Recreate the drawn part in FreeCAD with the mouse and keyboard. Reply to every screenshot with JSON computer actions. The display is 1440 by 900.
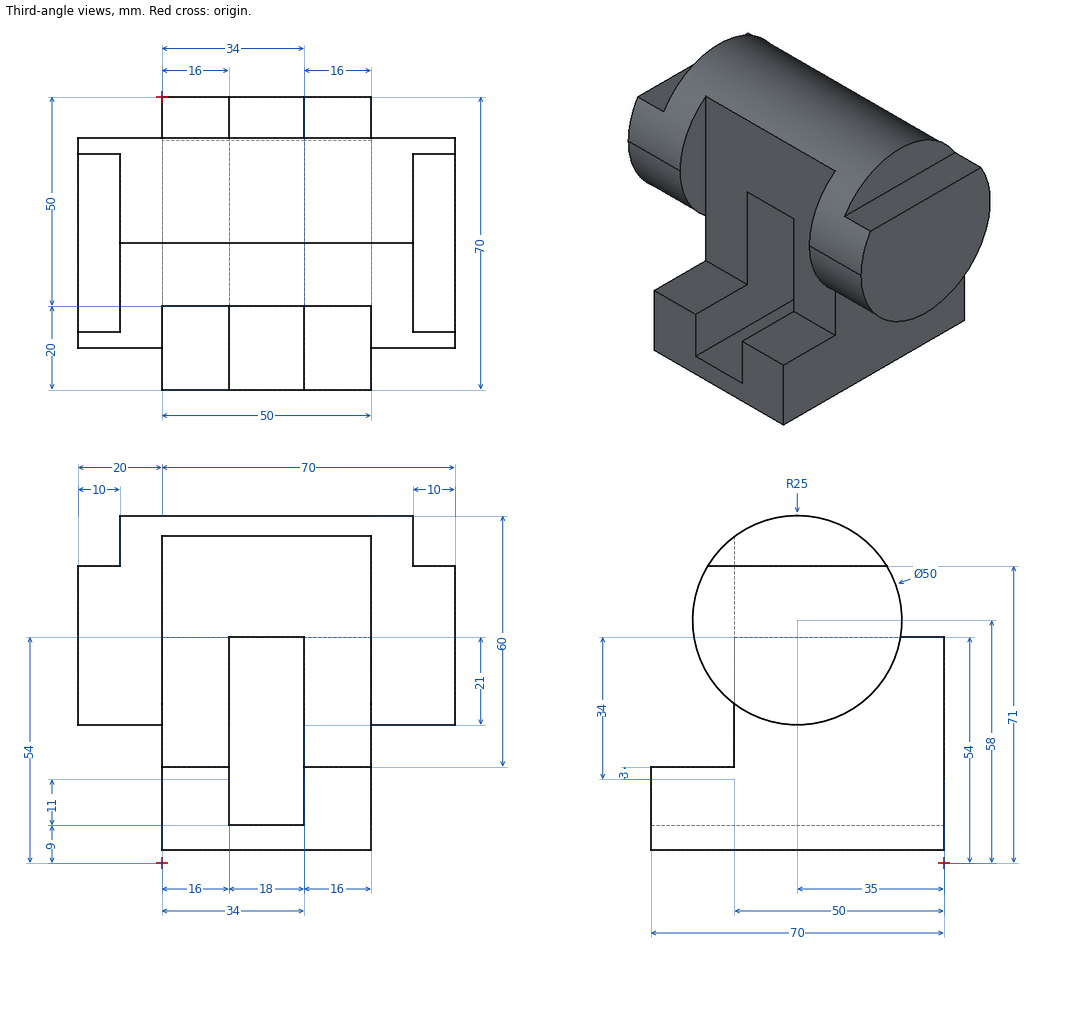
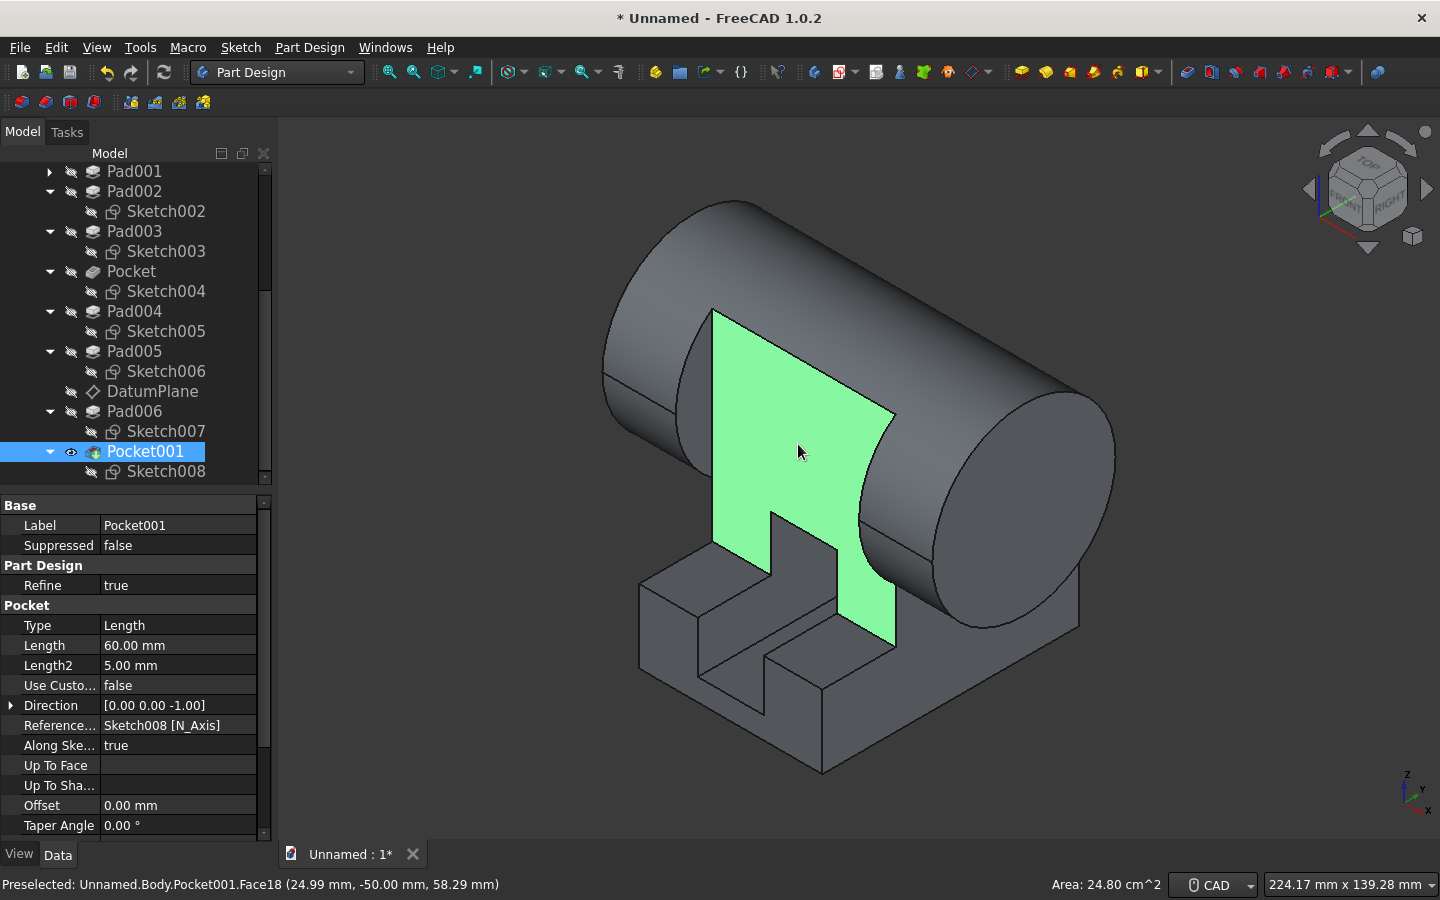
{"action": "left_click", "coordinate": [840, 72]}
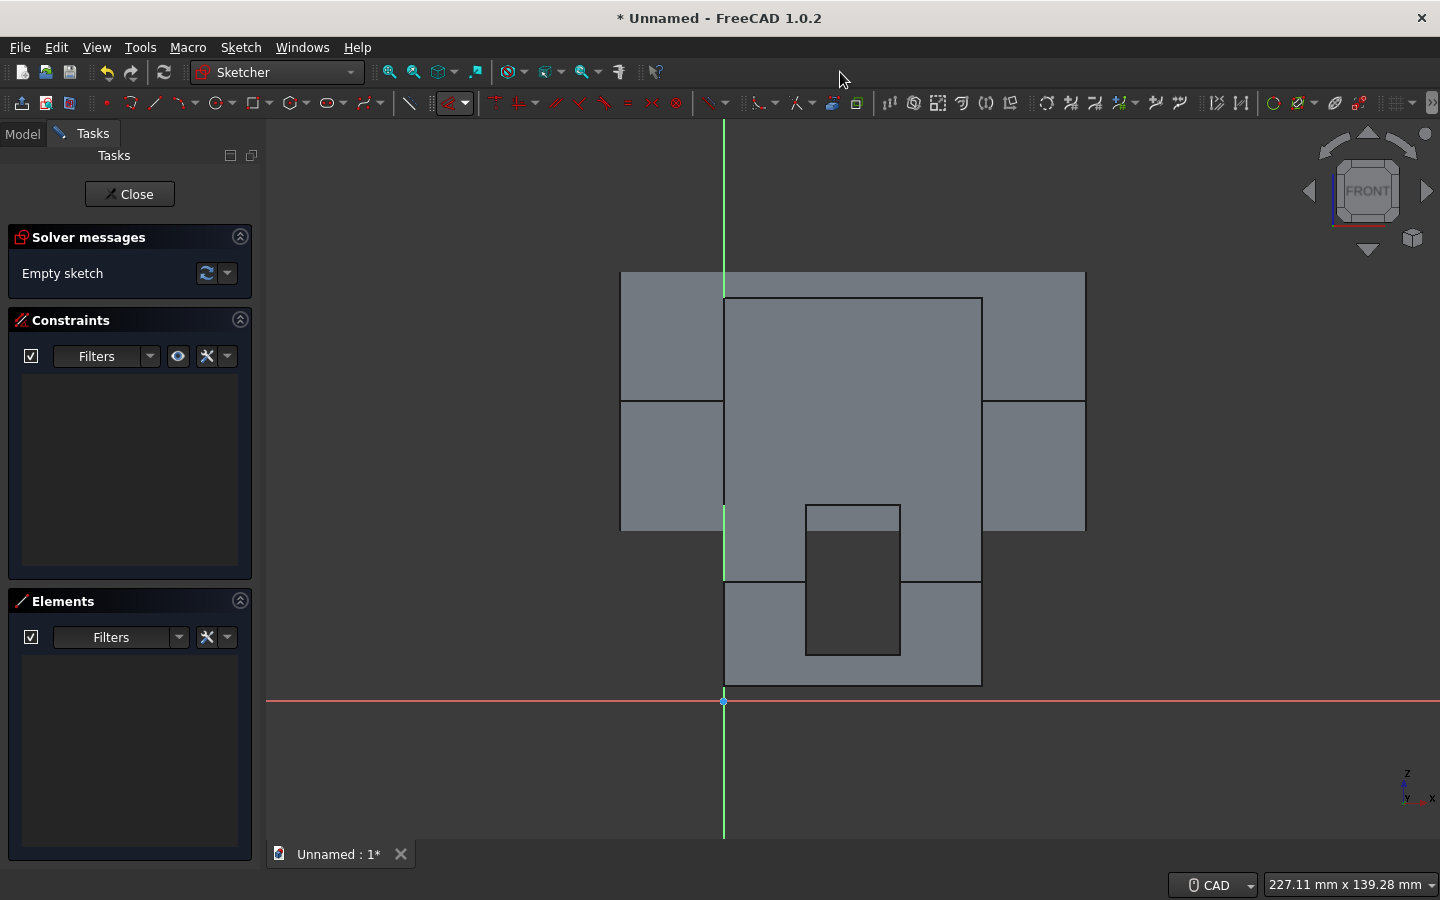
{"action": "key", "text": "q s"}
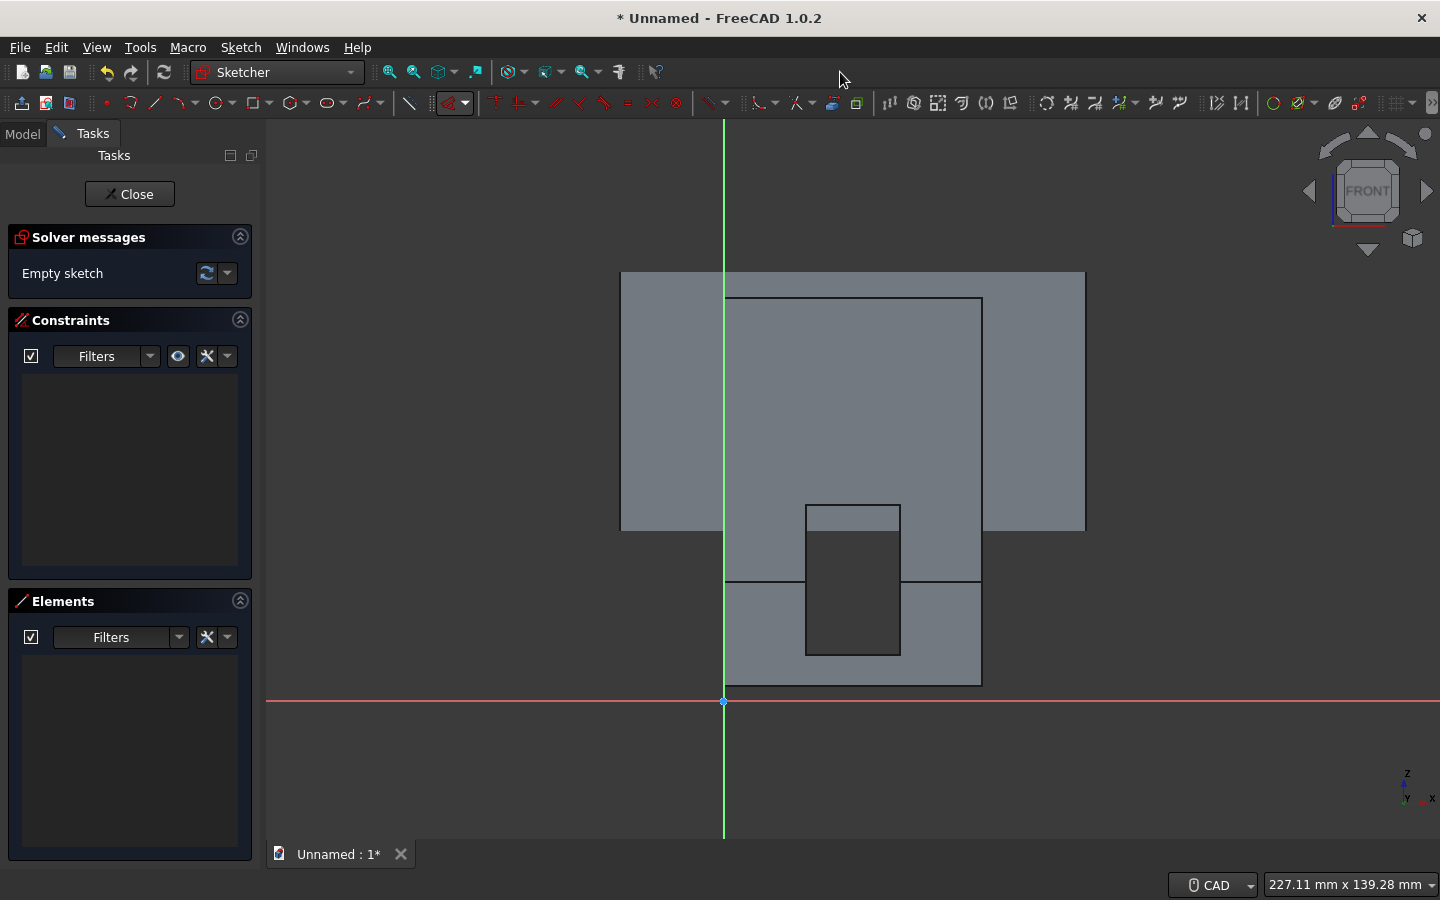
{"action": "scroll", "coordinate": [875, 476], "scroll_direction": "up", "scroll_amount": 7}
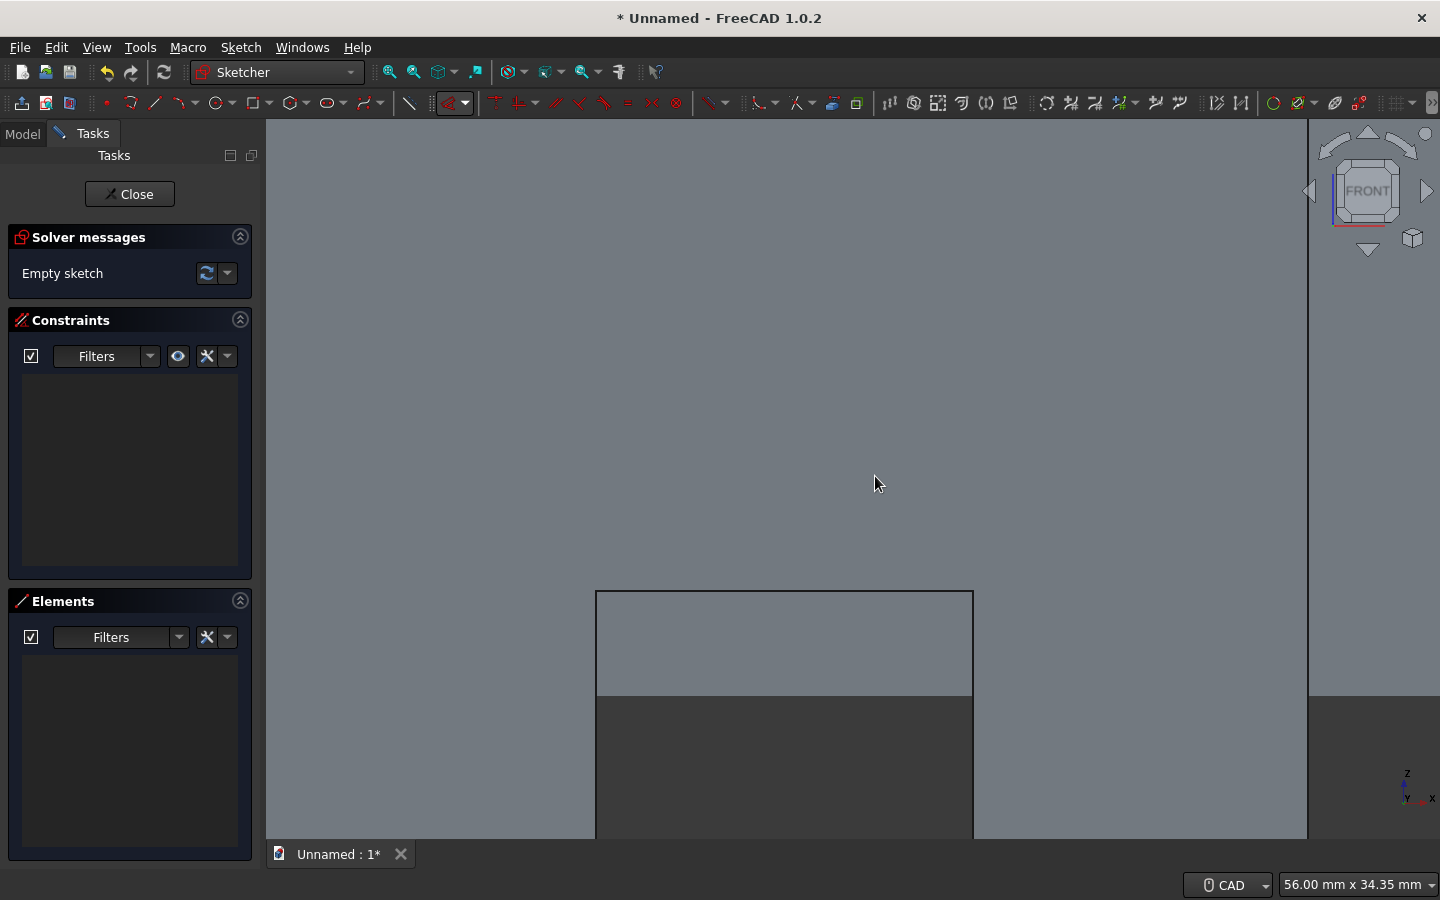
{"action": "key", "text": "g r"}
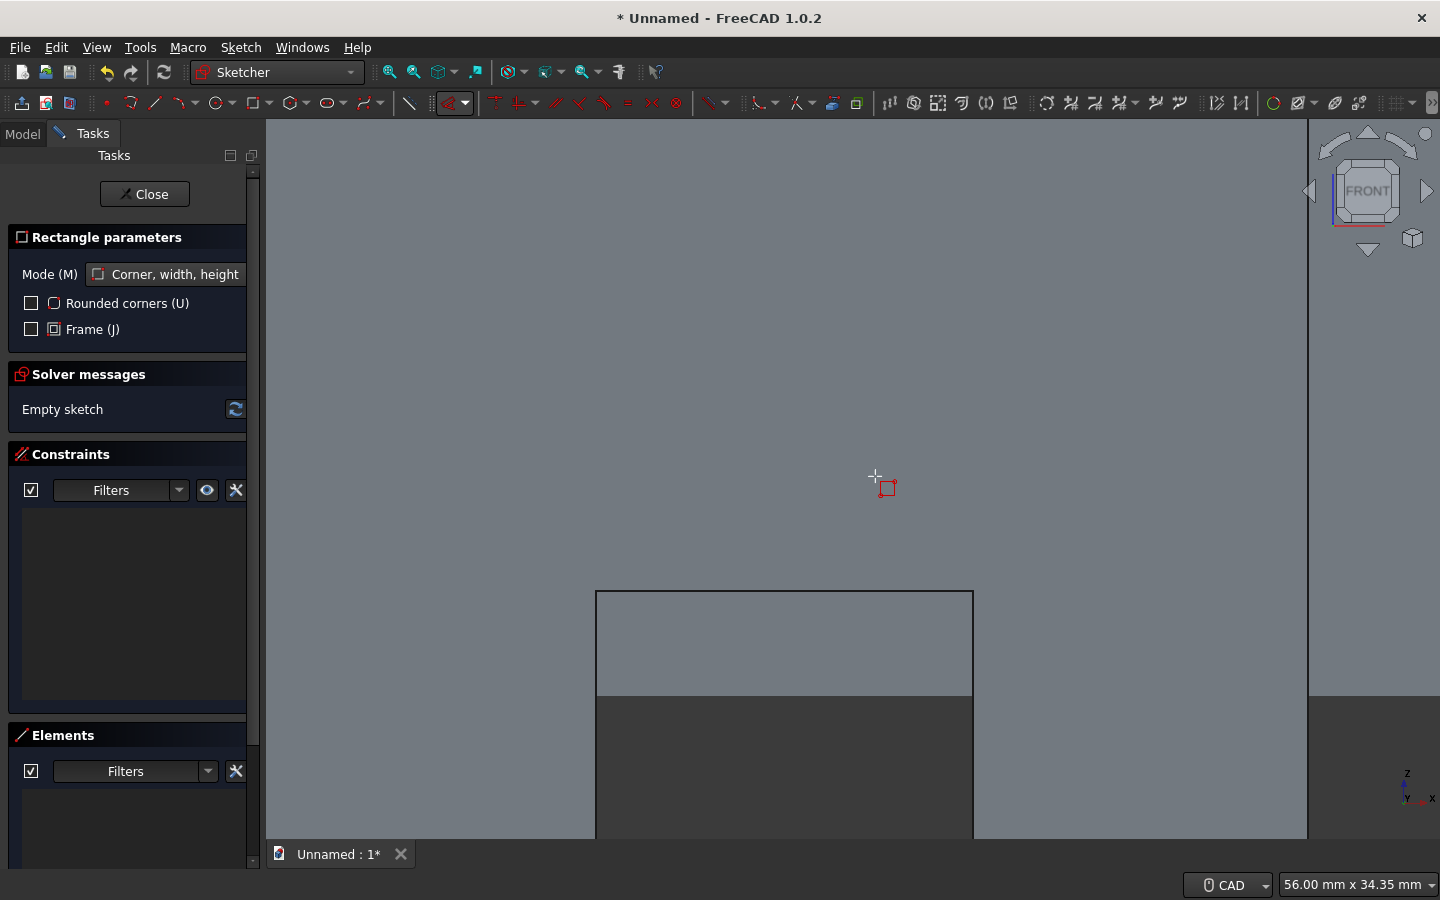
{"action": "left_click", "coordinate": [596, 256]}
{"action": "mouse_move", "coordinate": [973, 696]}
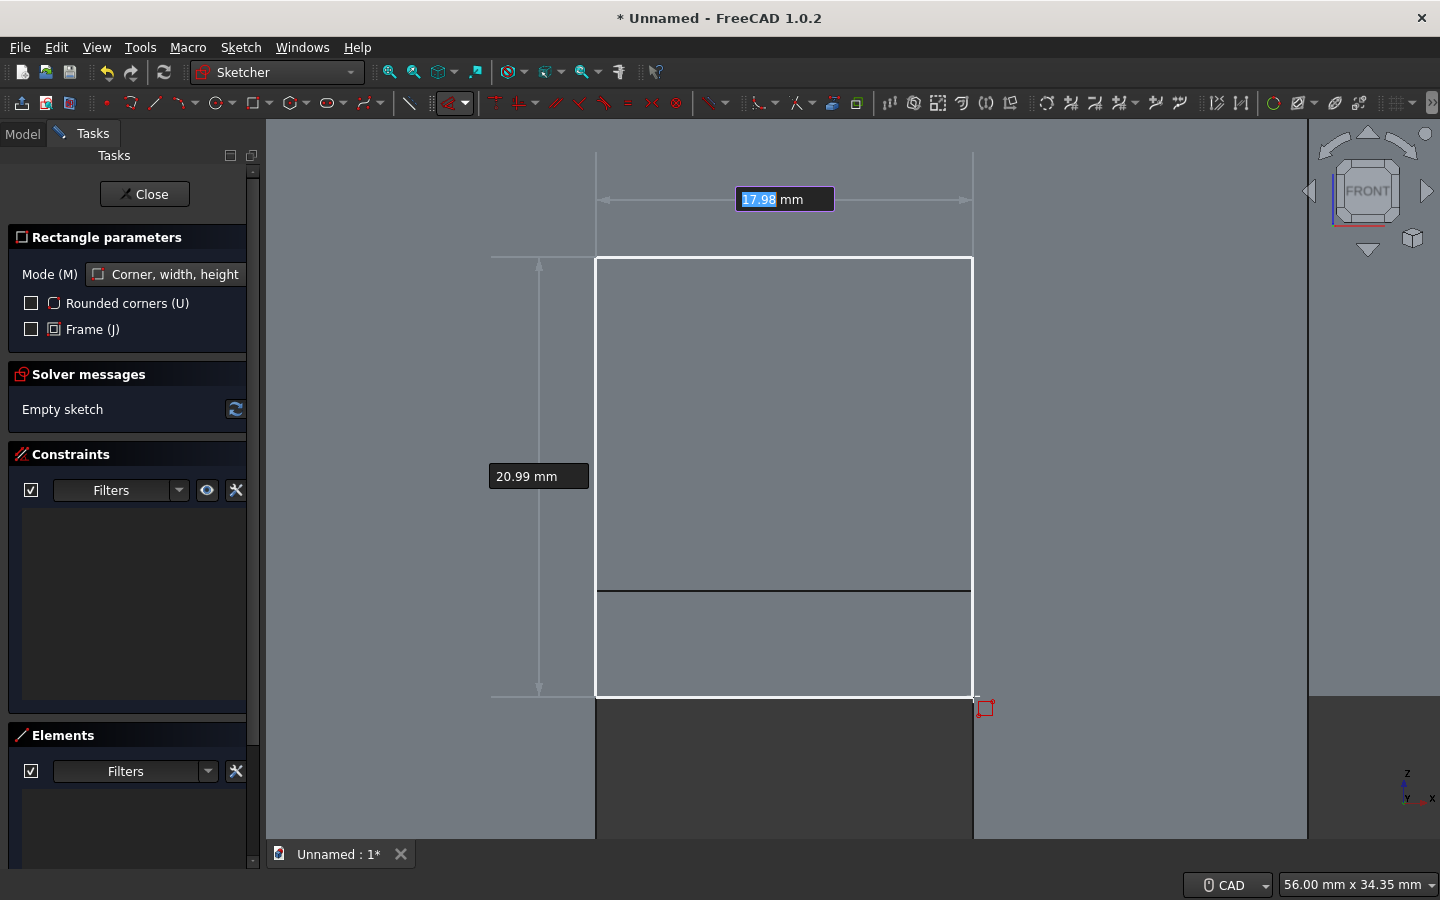
{"action": "type", "text": "18"}
{"action": "key", "text": "Tab"}
{"action": "type", "text": "21"}
{"action": "key", "text": "Return"}
{"action": "key", "text": "Escape"}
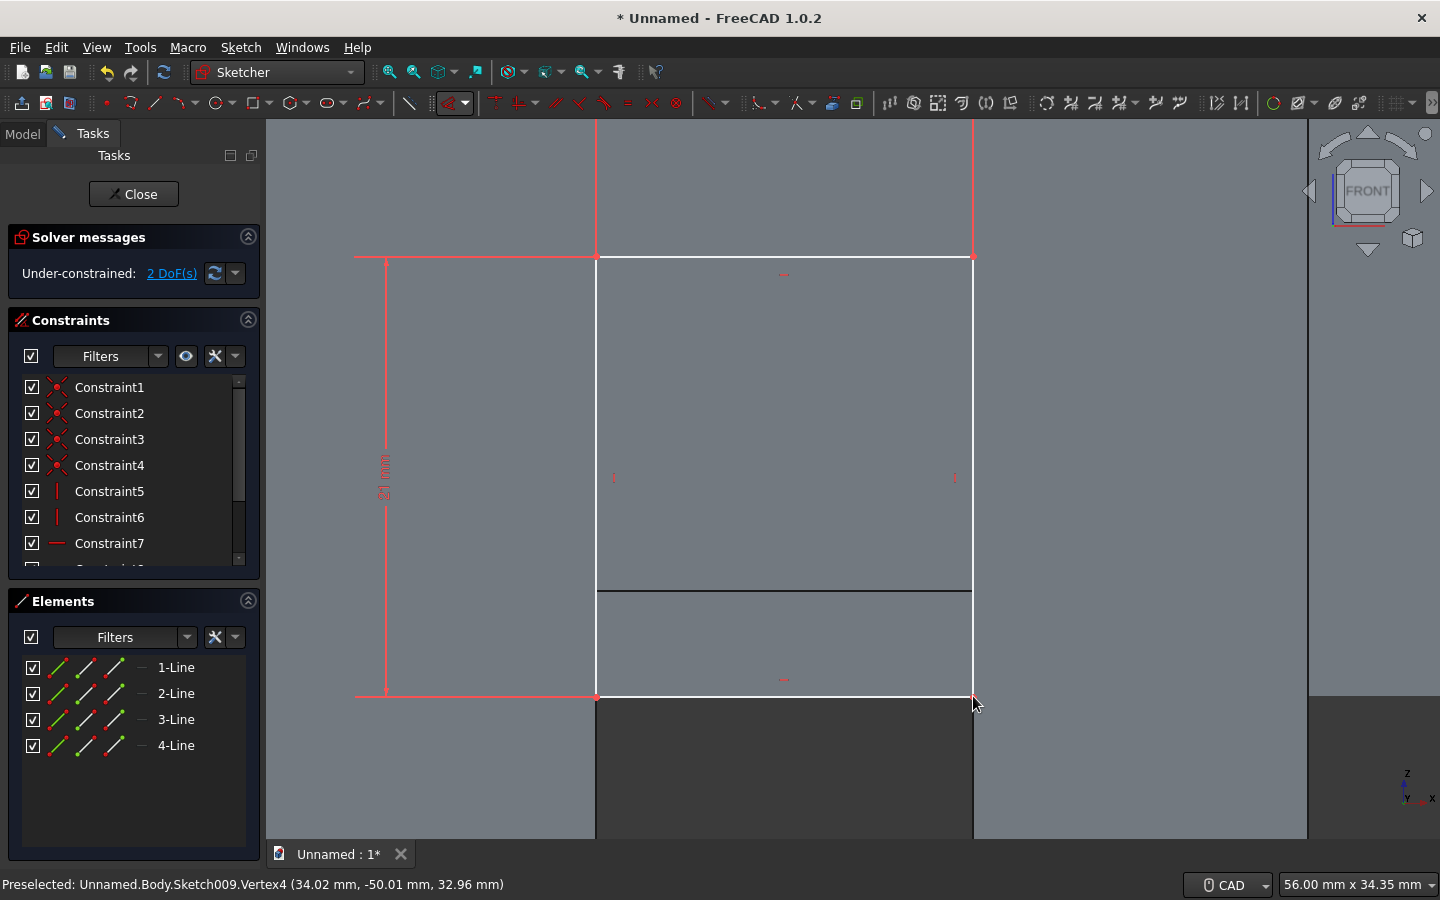
{"action": "left_click", "coordinate": [596, 257]}